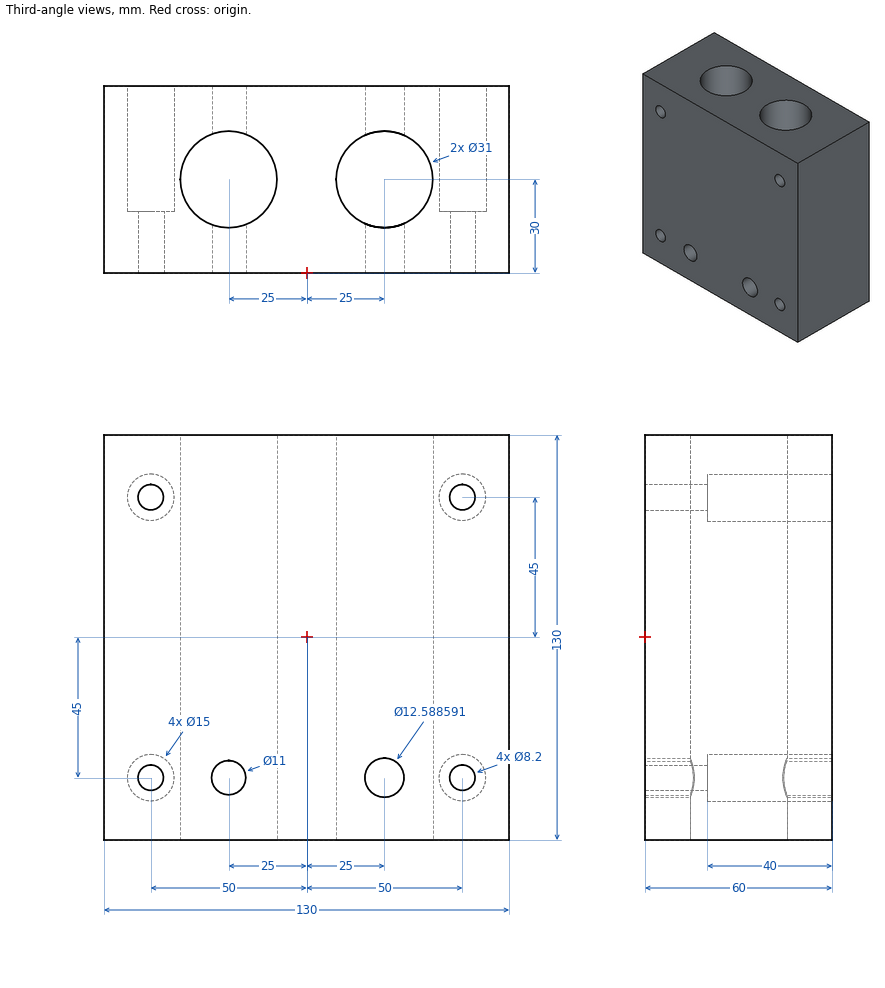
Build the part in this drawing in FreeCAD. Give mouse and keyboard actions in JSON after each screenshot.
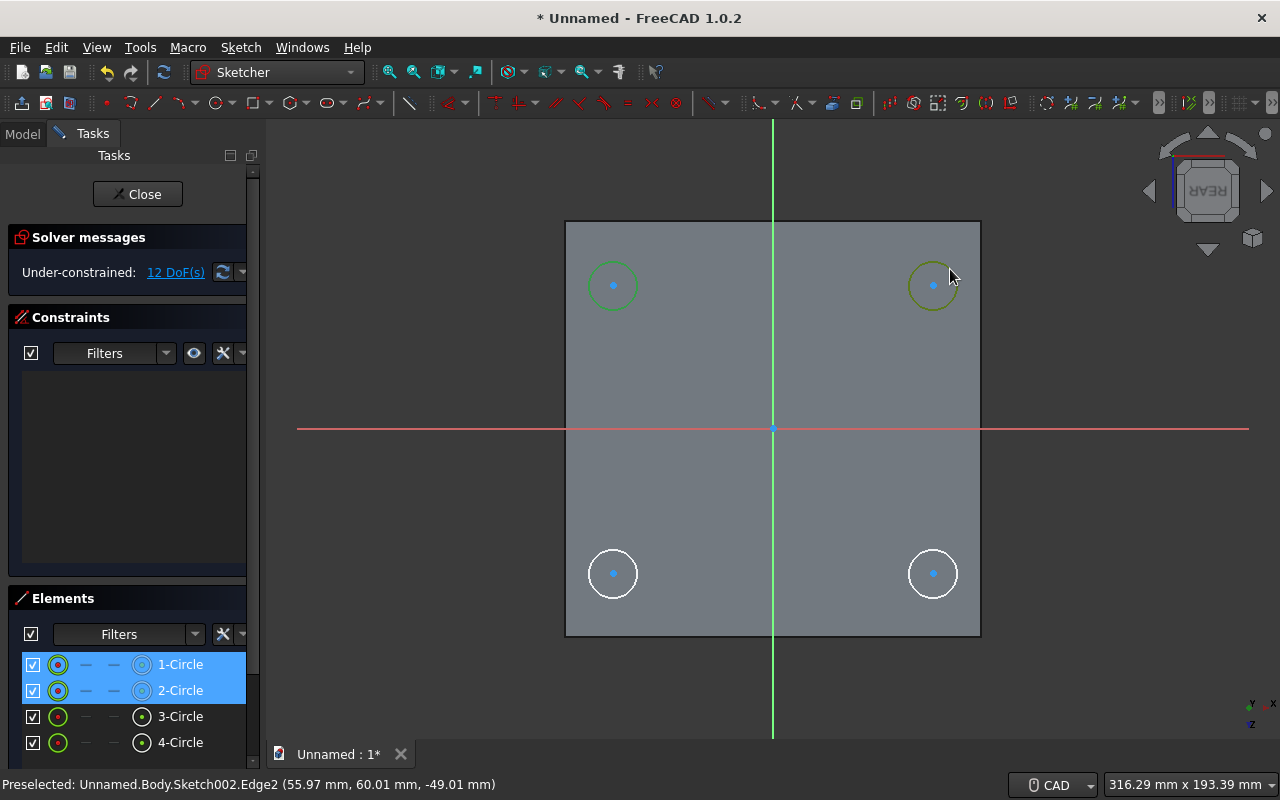
{"action": "left_click", "coordinate": [950, 557]}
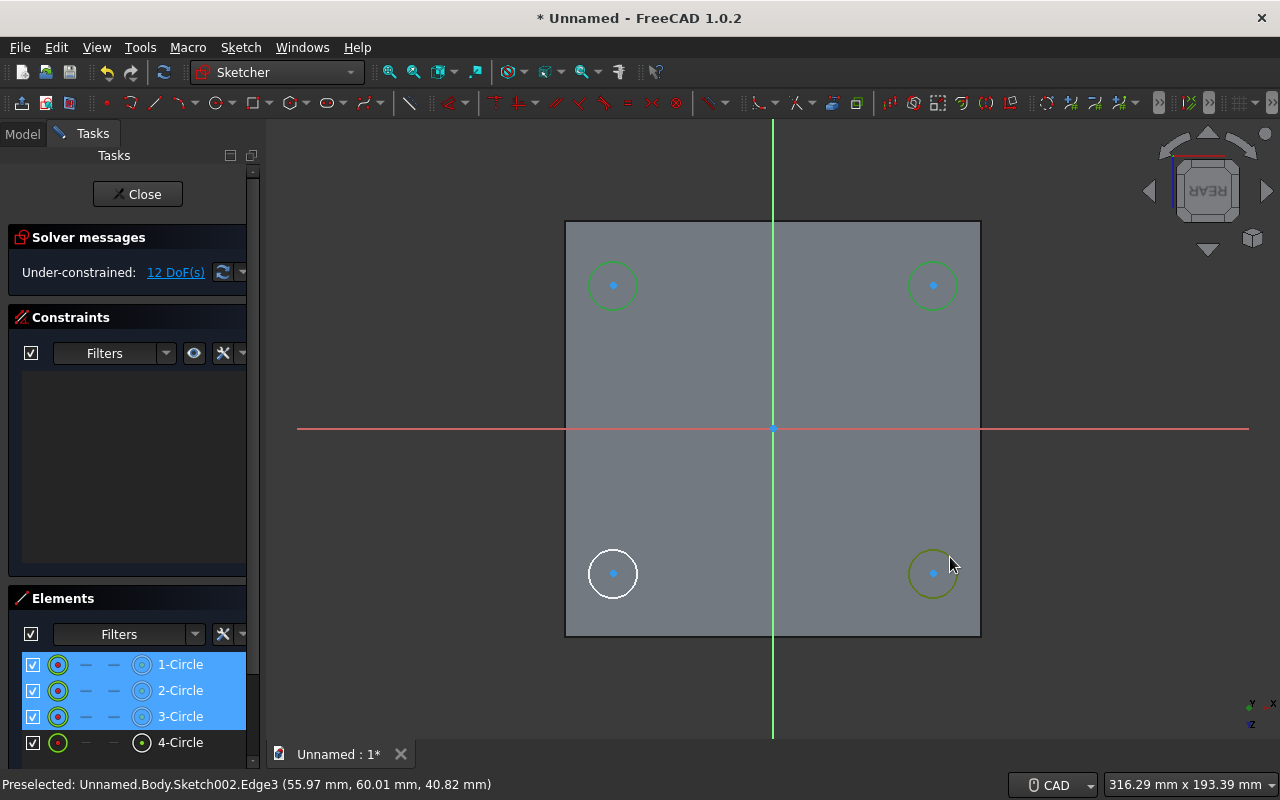
{"action": "left_click", "coordinate": [630, 557]}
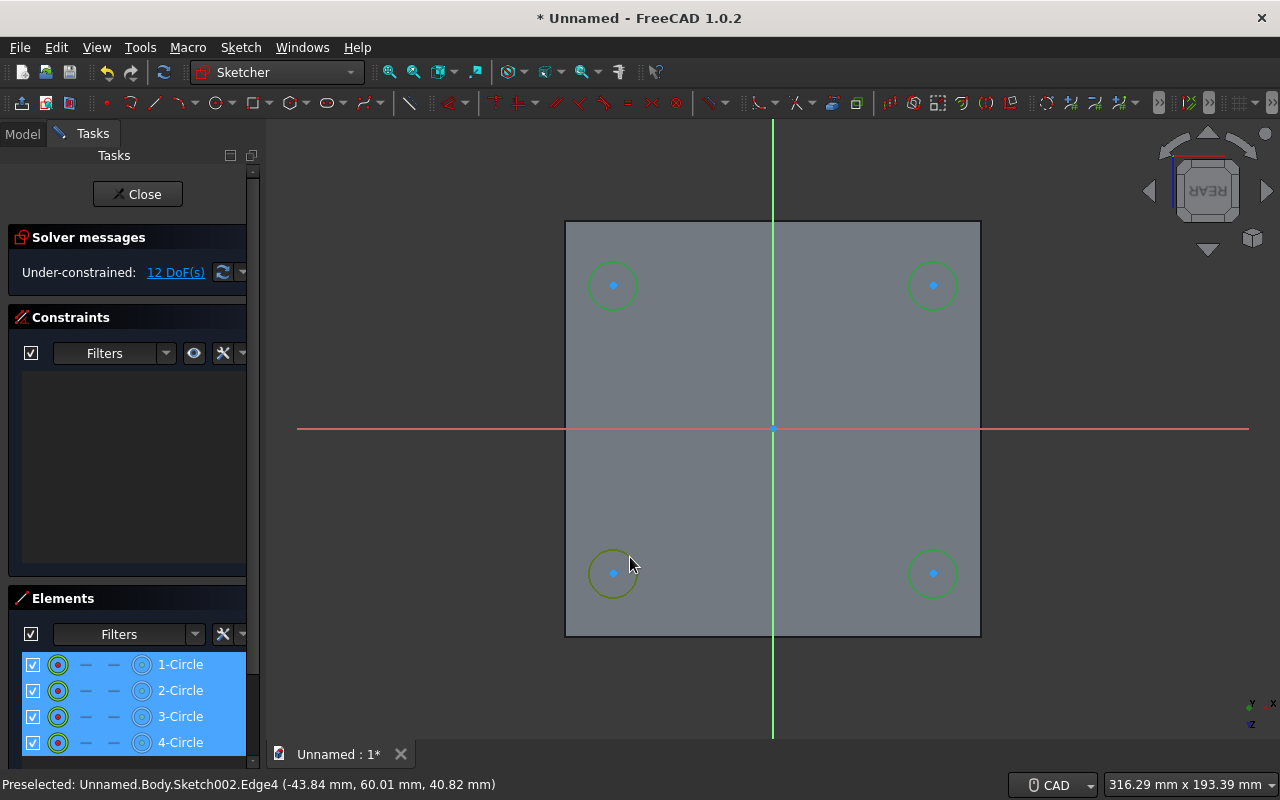
{"action": "key", "text": "e"}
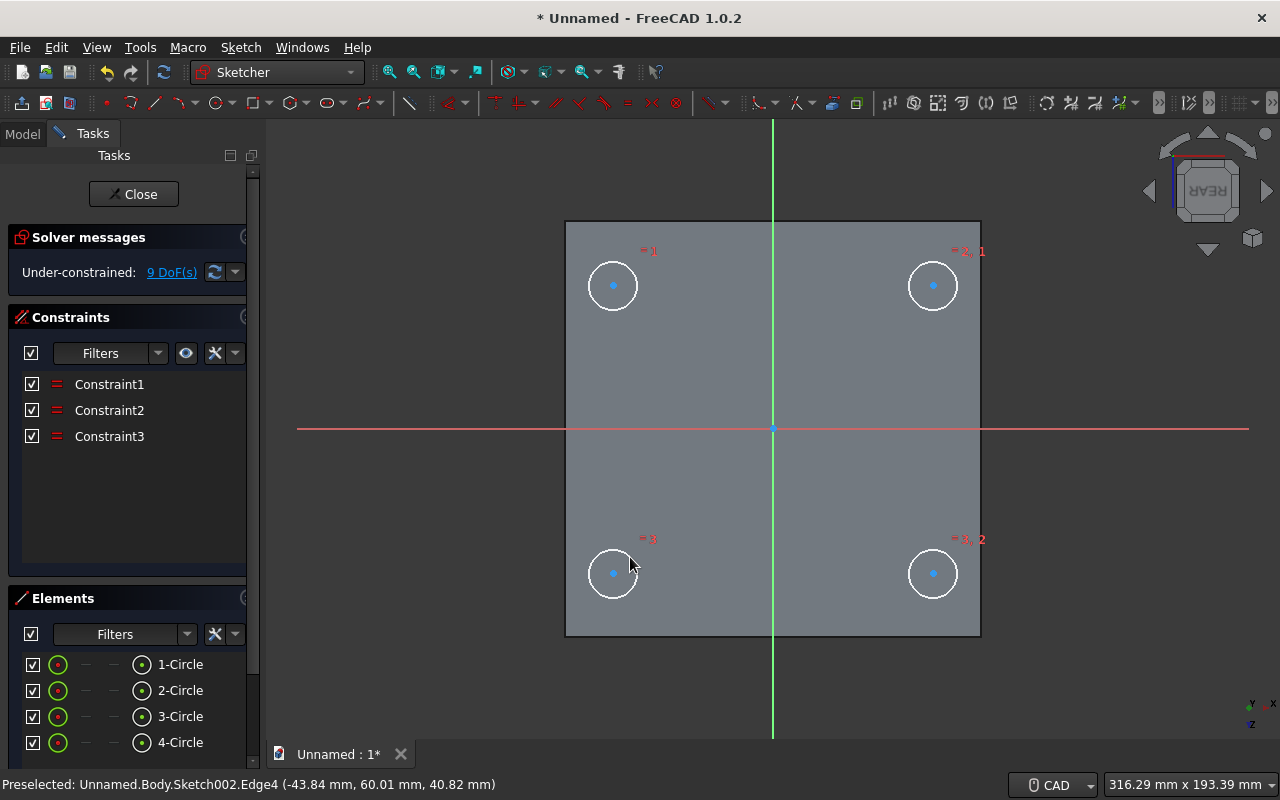
{"action": "left_click", "coordinate": [613, 286]}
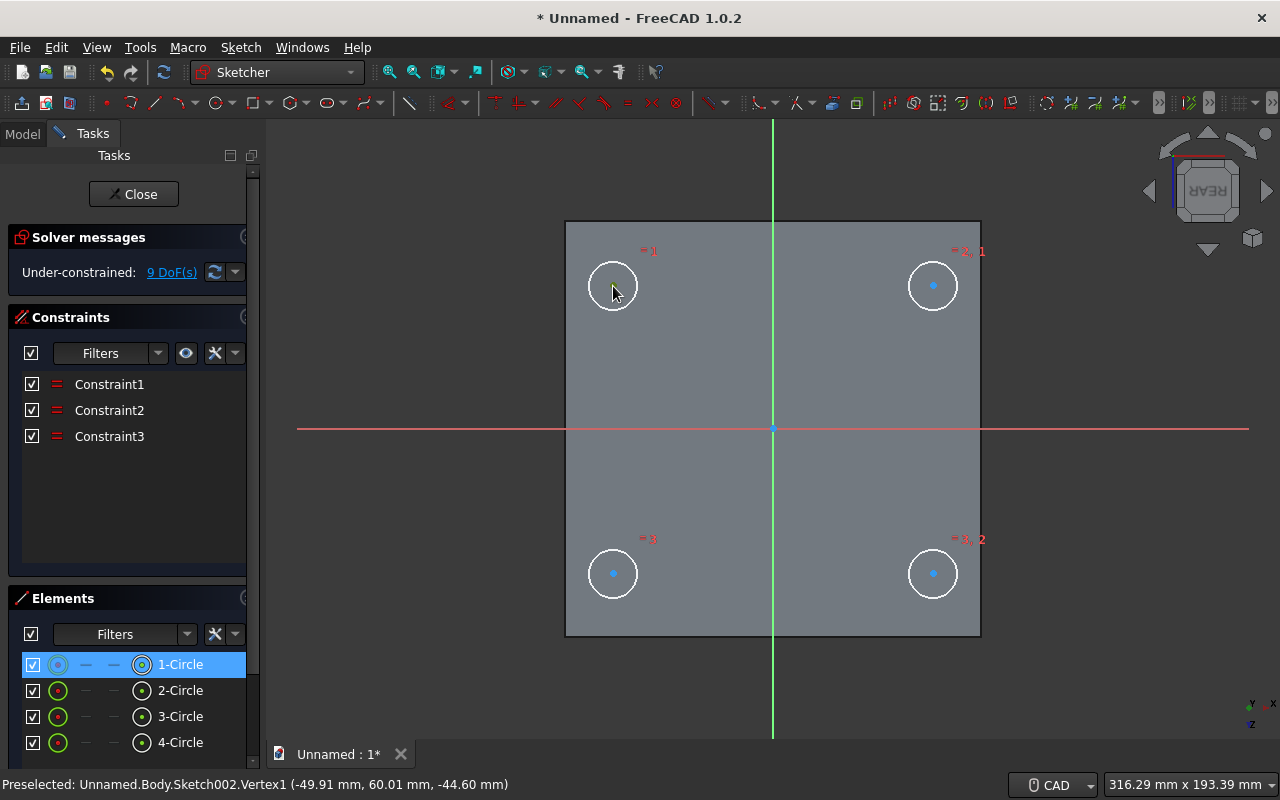
{"action": "left_click", "coordinate": [933, 286]}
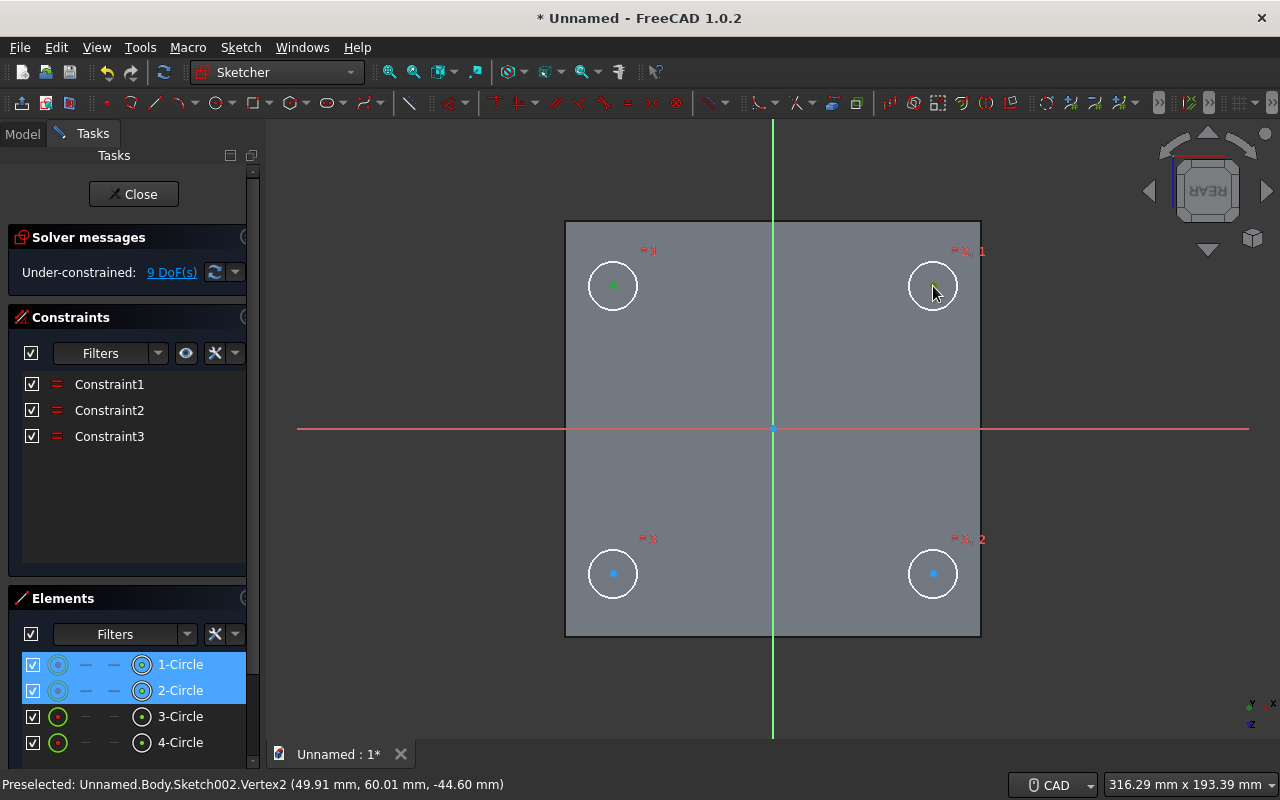
{"action": "key", "text": "h"}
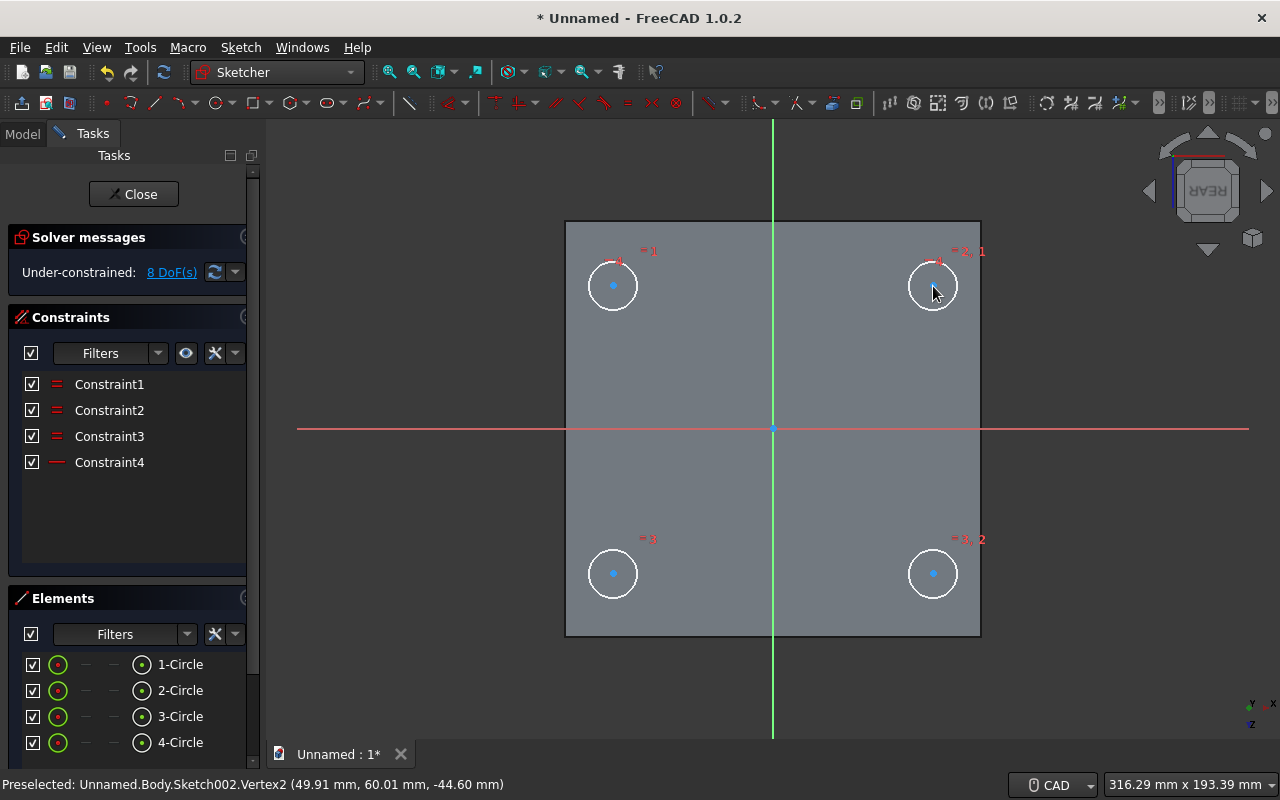
{"action": "left_click", "coordinate": [933, 286]}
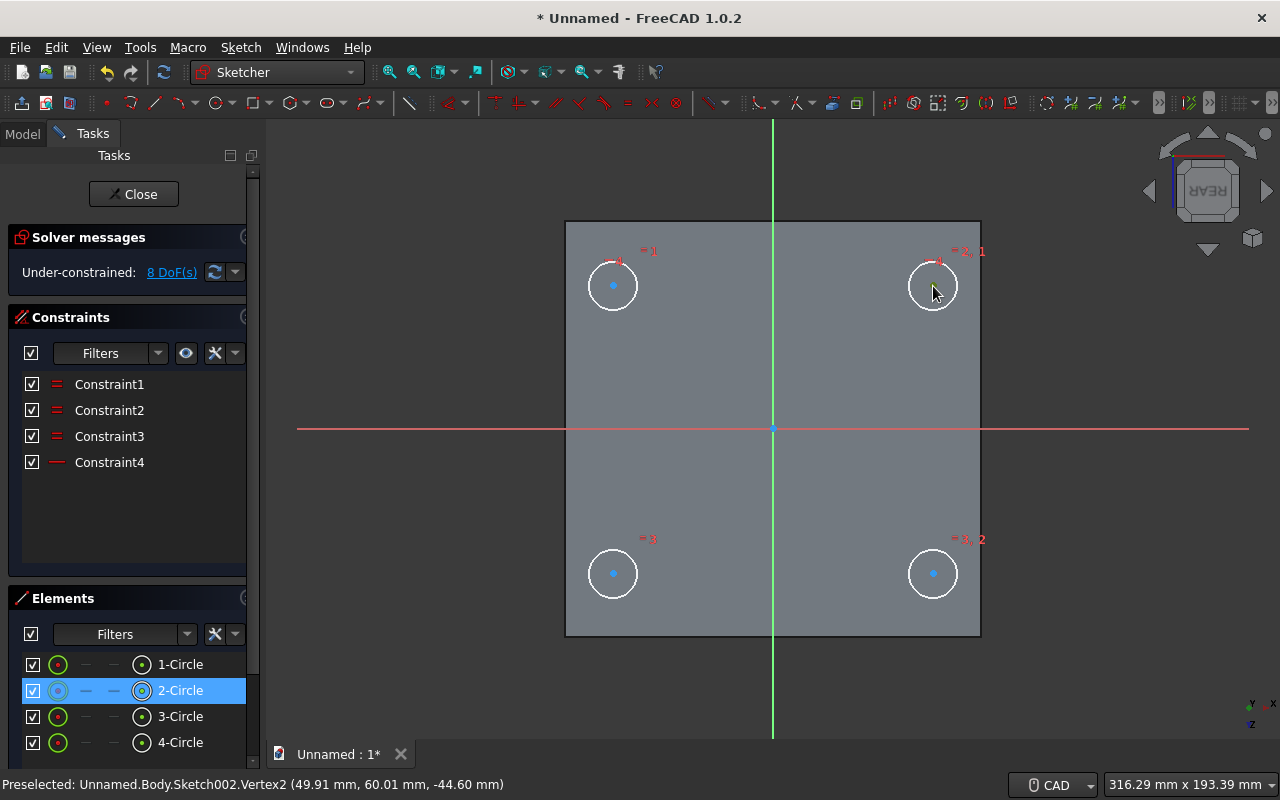
{"action": "left_click", "coordinate": [933, 574]}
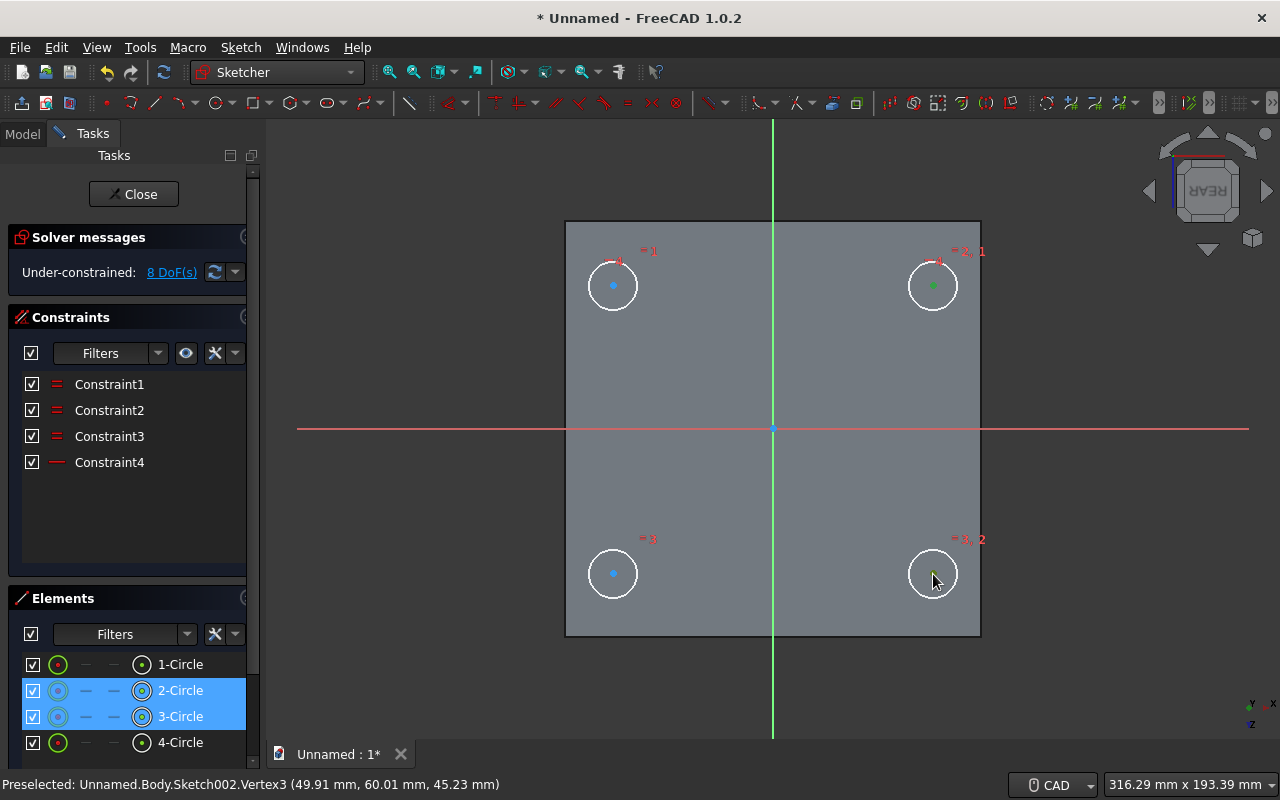
{"action": "key", "text": "v"}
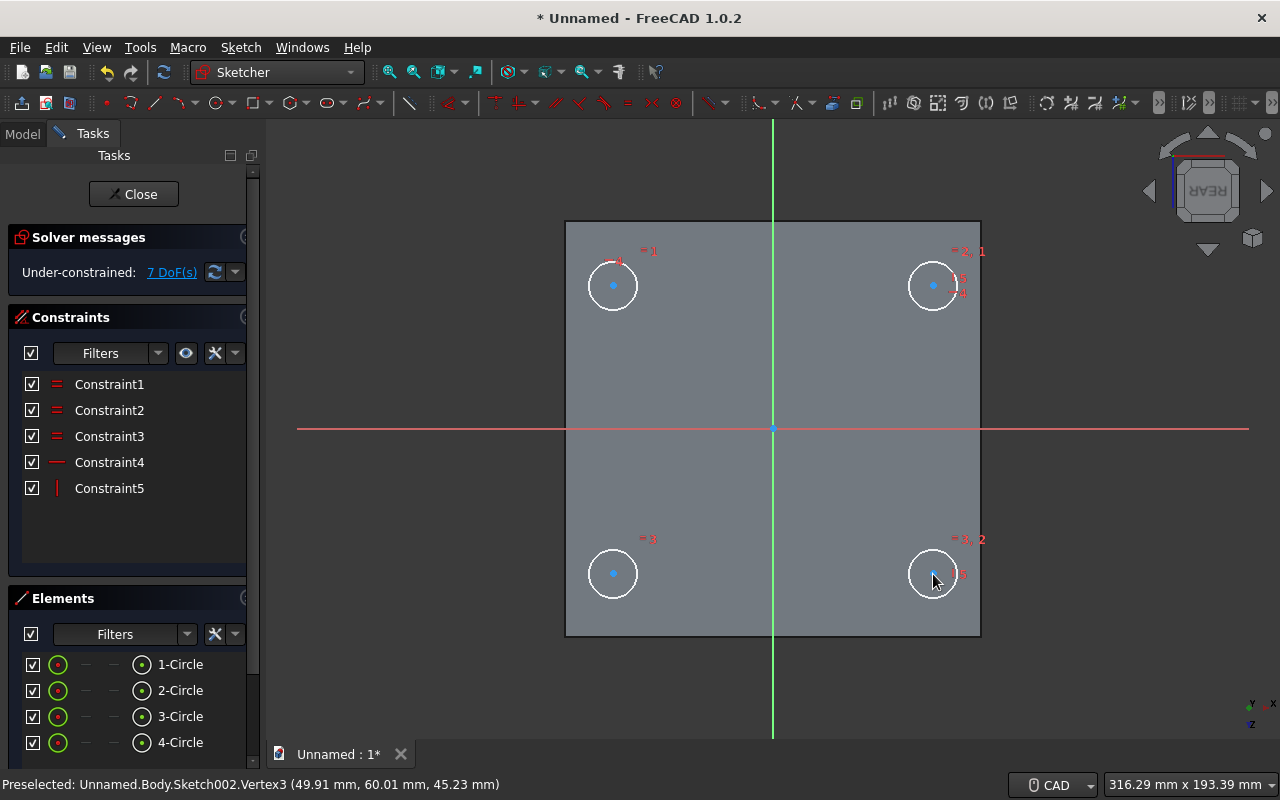
{"action": "left_click", "coordinate": [613, 286]}